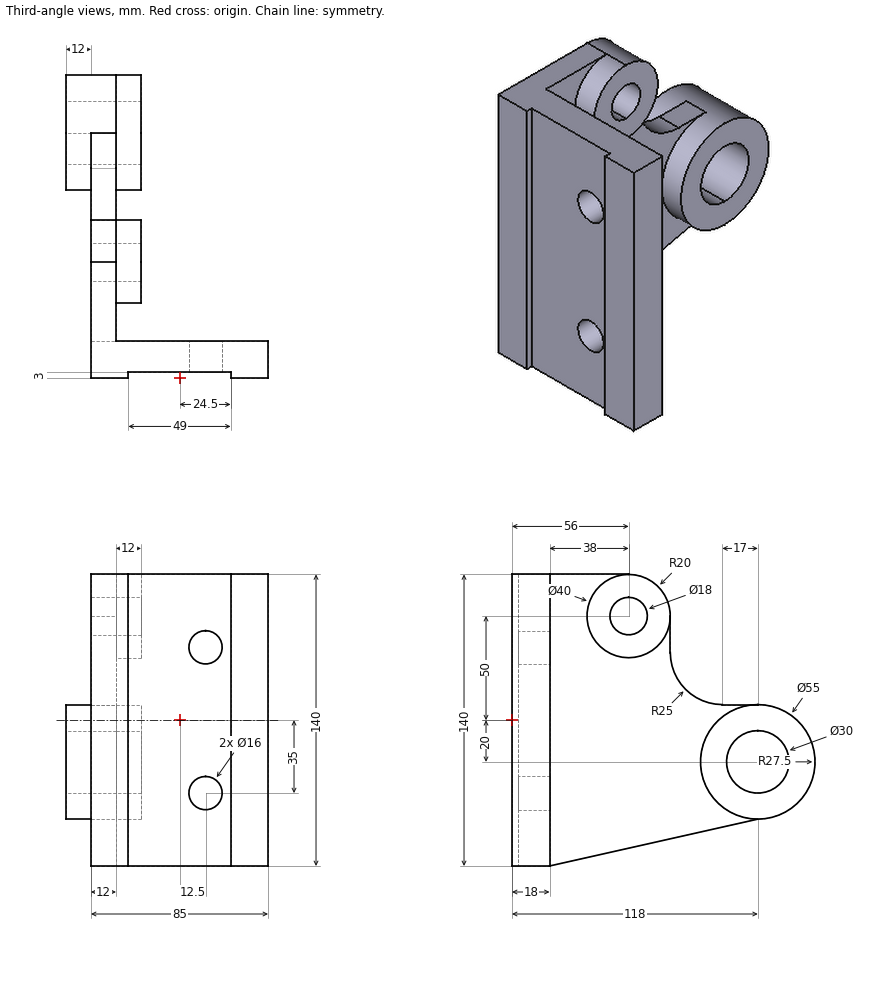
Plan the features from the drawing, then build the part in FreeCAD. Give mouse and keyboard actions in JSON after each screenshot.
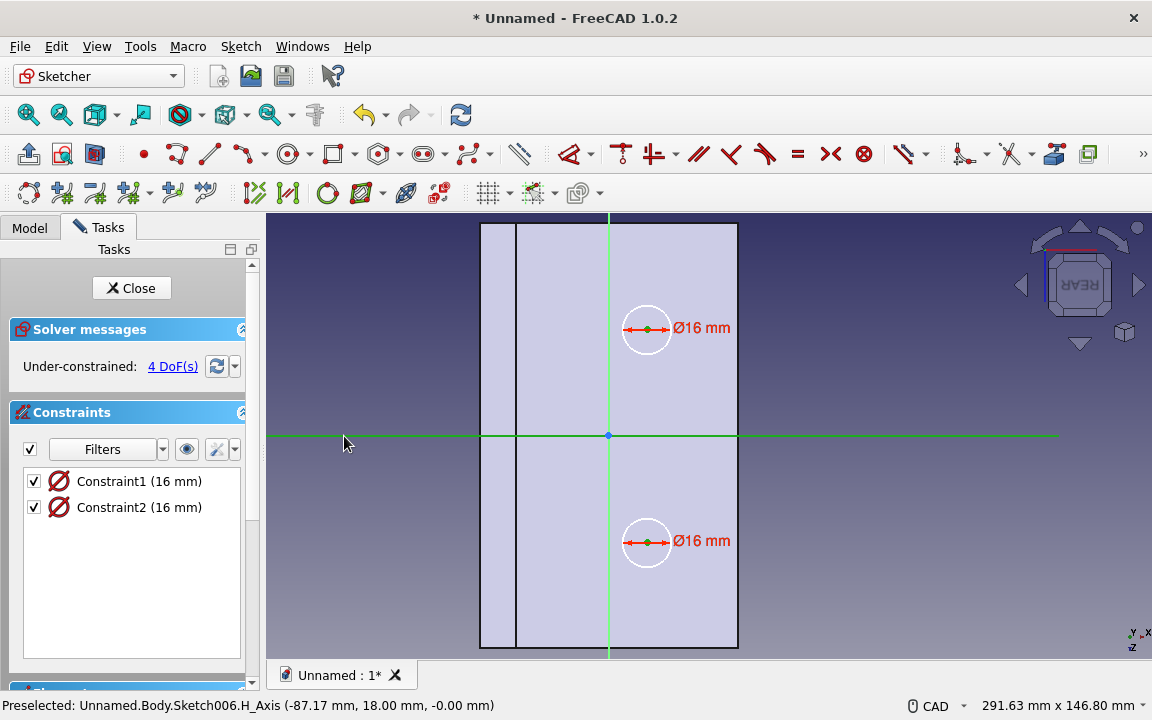
{"action": "key", "text": "s"}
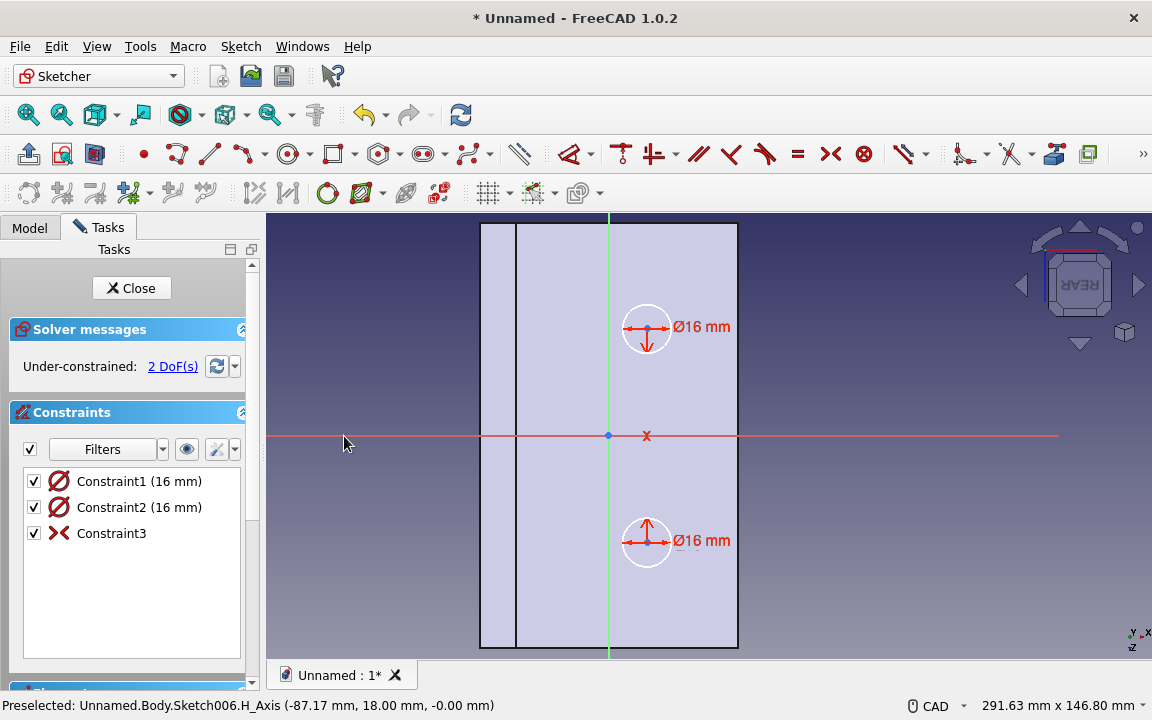
{"action": "key", "text": "d"}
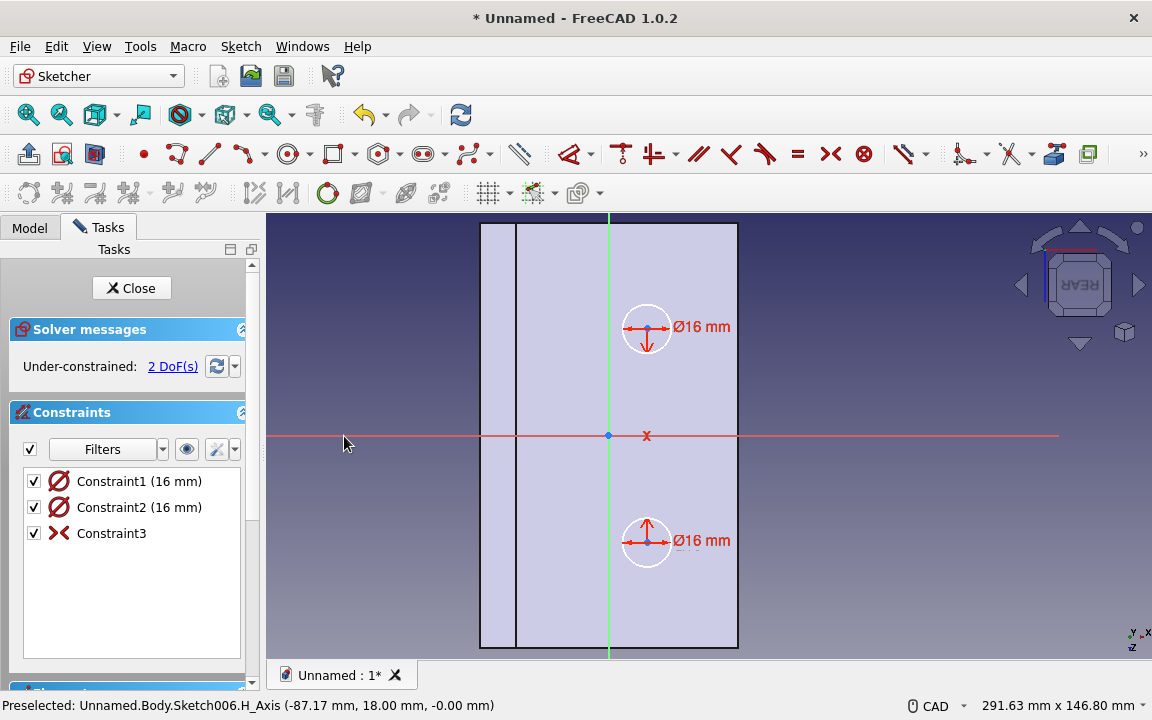
{"action": "left_click", "coordinate": [647, 329]}
{"action": "left_click", "coordinate": [575, 382]}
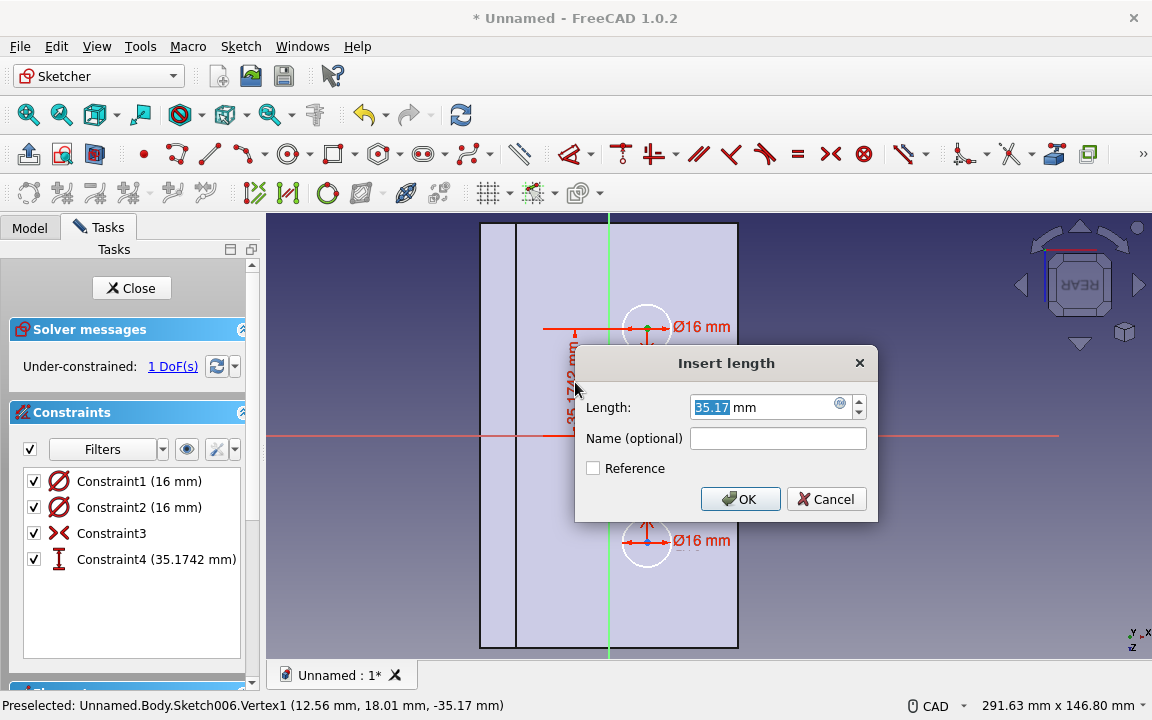
{"action": "type", "text": "35"}
{"action": "key", "text": "Return"}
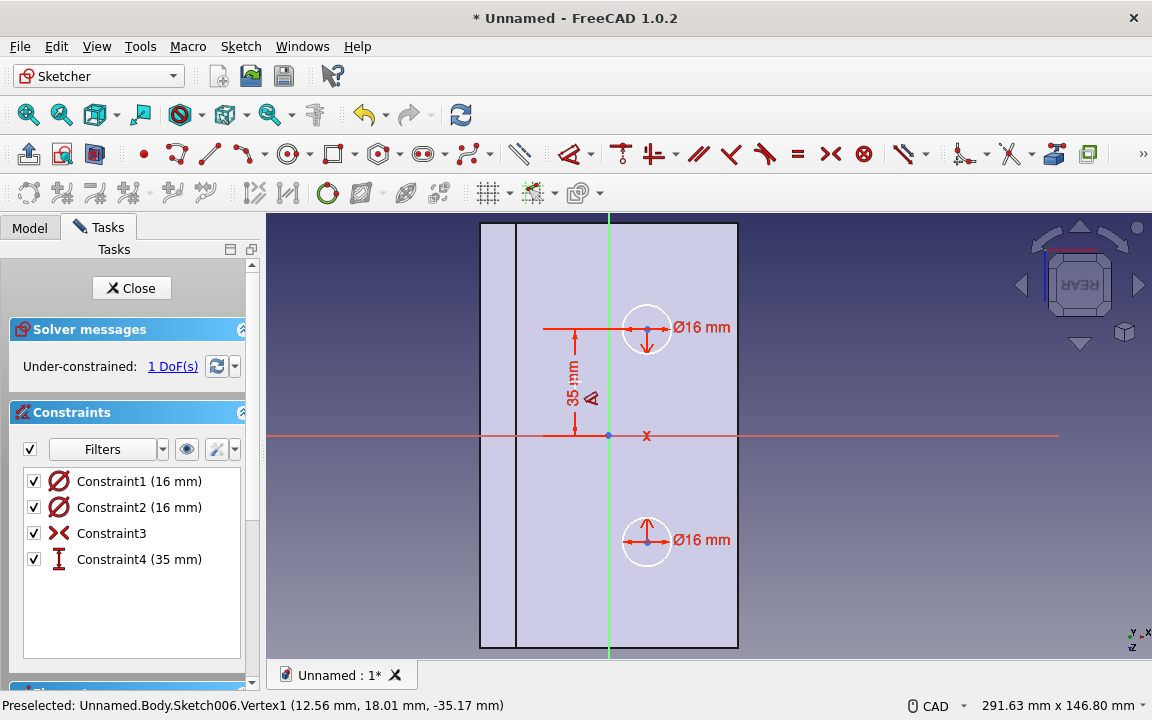
{"action": "left_click", "coordinate": [647, 329]}
{"action": "left_click", "coordinate": [628, 295]}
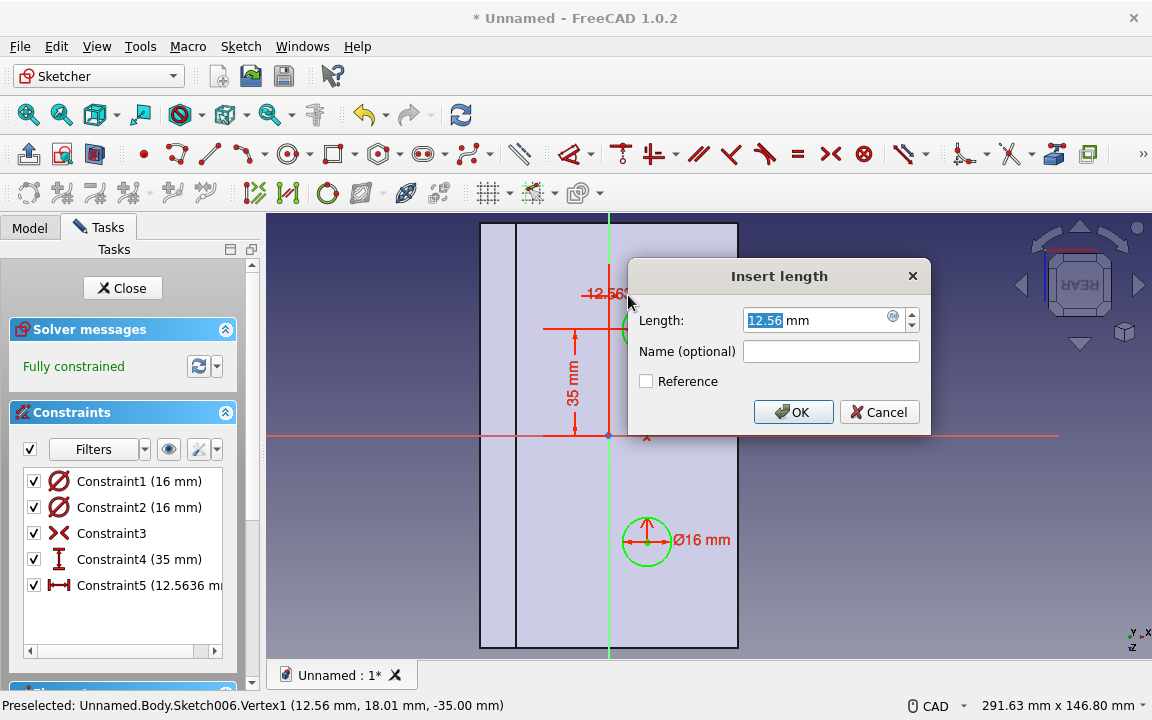
{"action": "type", "text": "12.5"}
{"action": "key", "text": "Return"}
{"action": "key", "text": "Escape"}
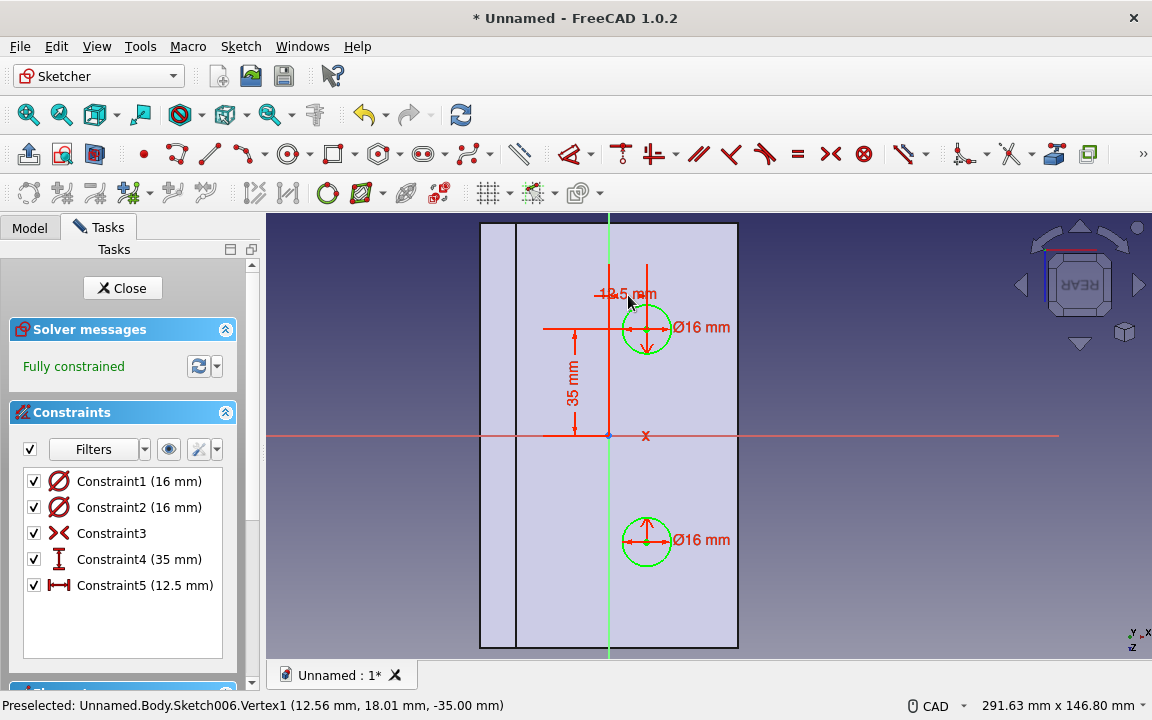
{"action": "left_click", "coordinate": [123, 288]}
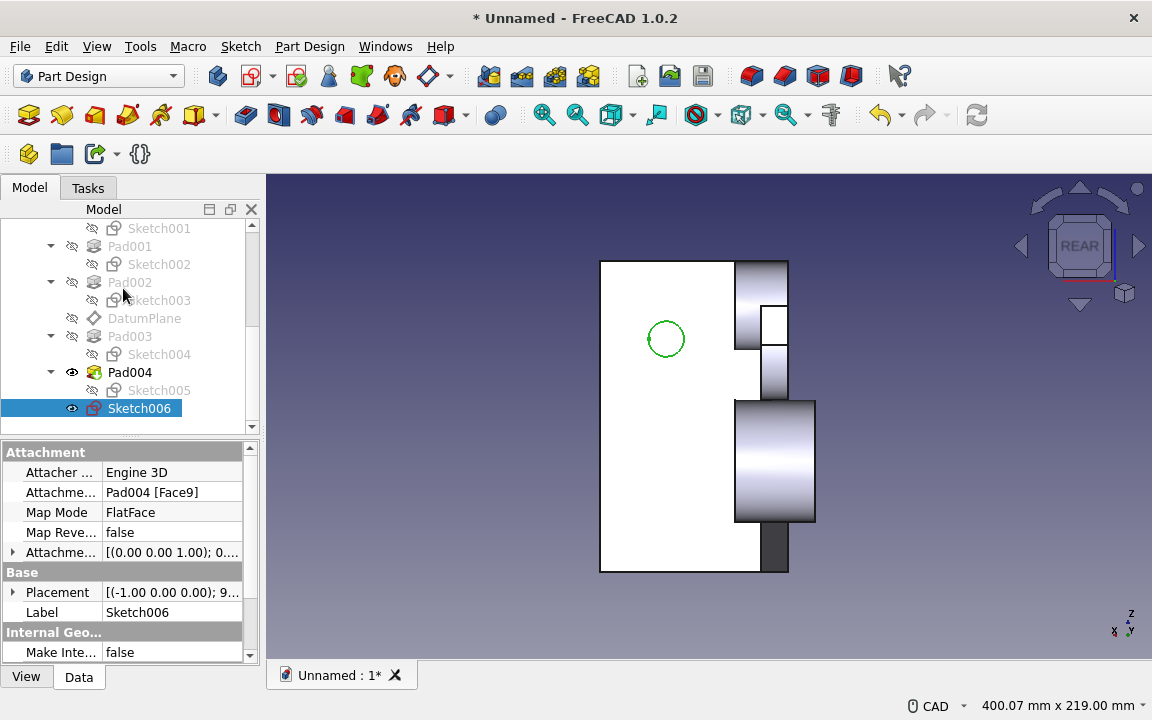
{"action": "left_click", "coordinate": [246, 116]}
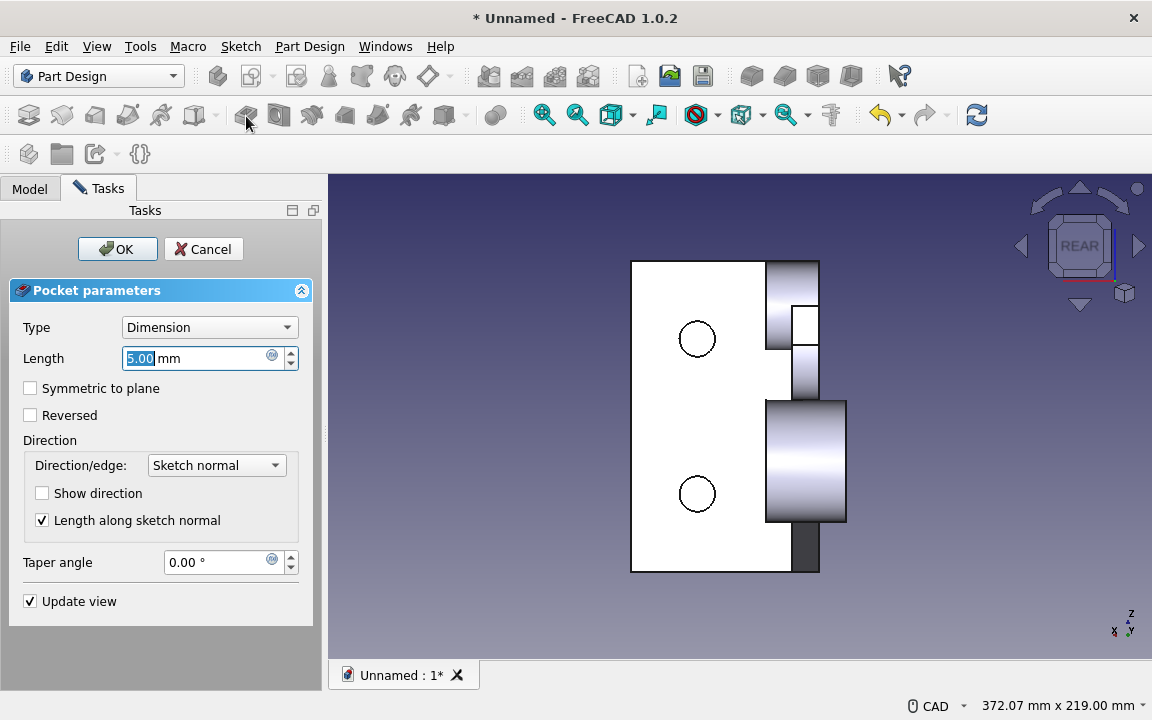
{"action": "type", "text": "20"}
{"action": "key", "text": "Tab"}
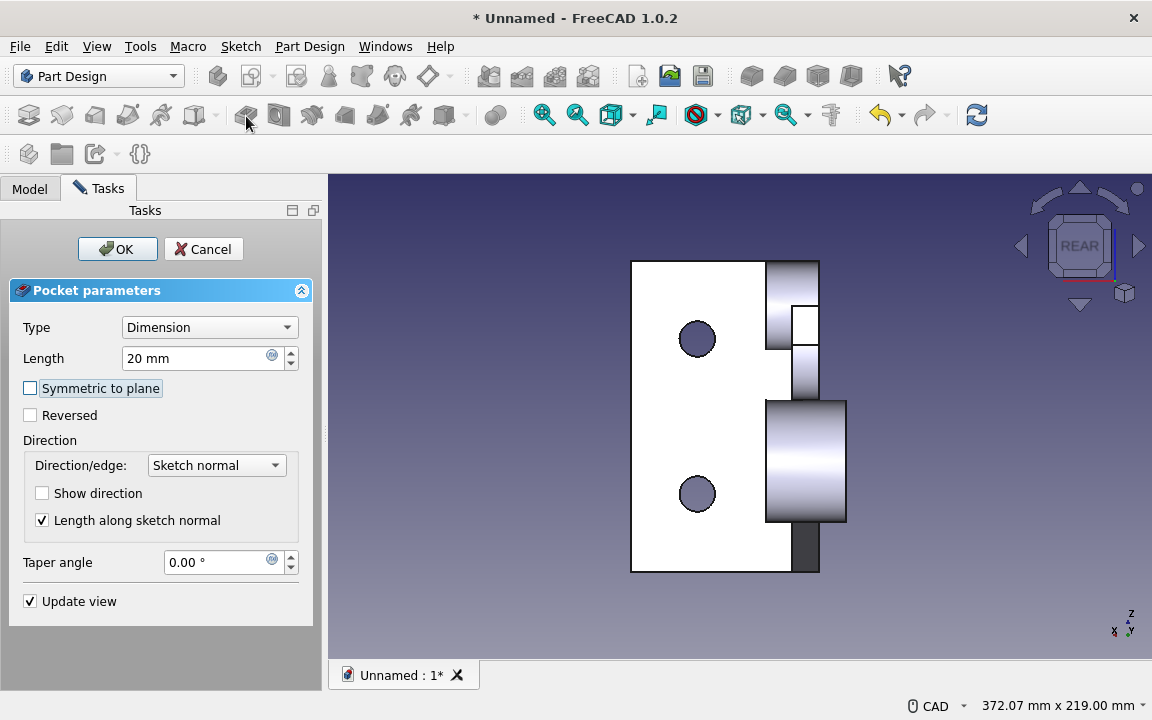
{"action": "left_click", "coordinate": [118, 249]}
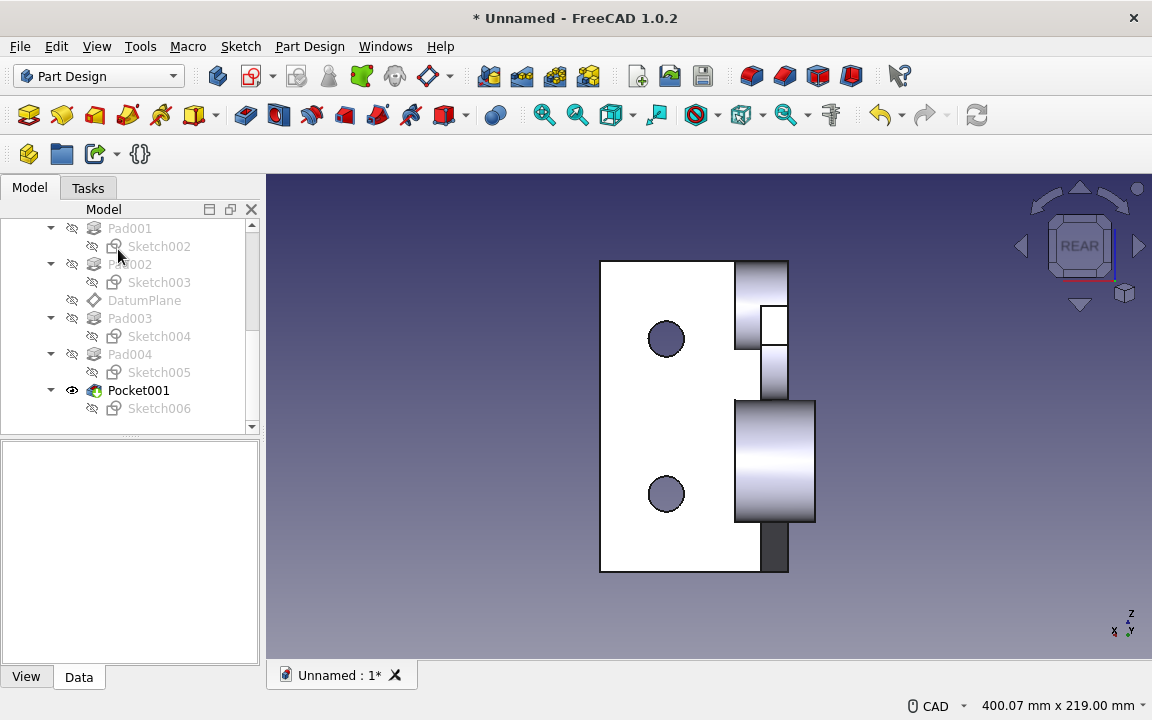
{"action": "key", "text": "0"}